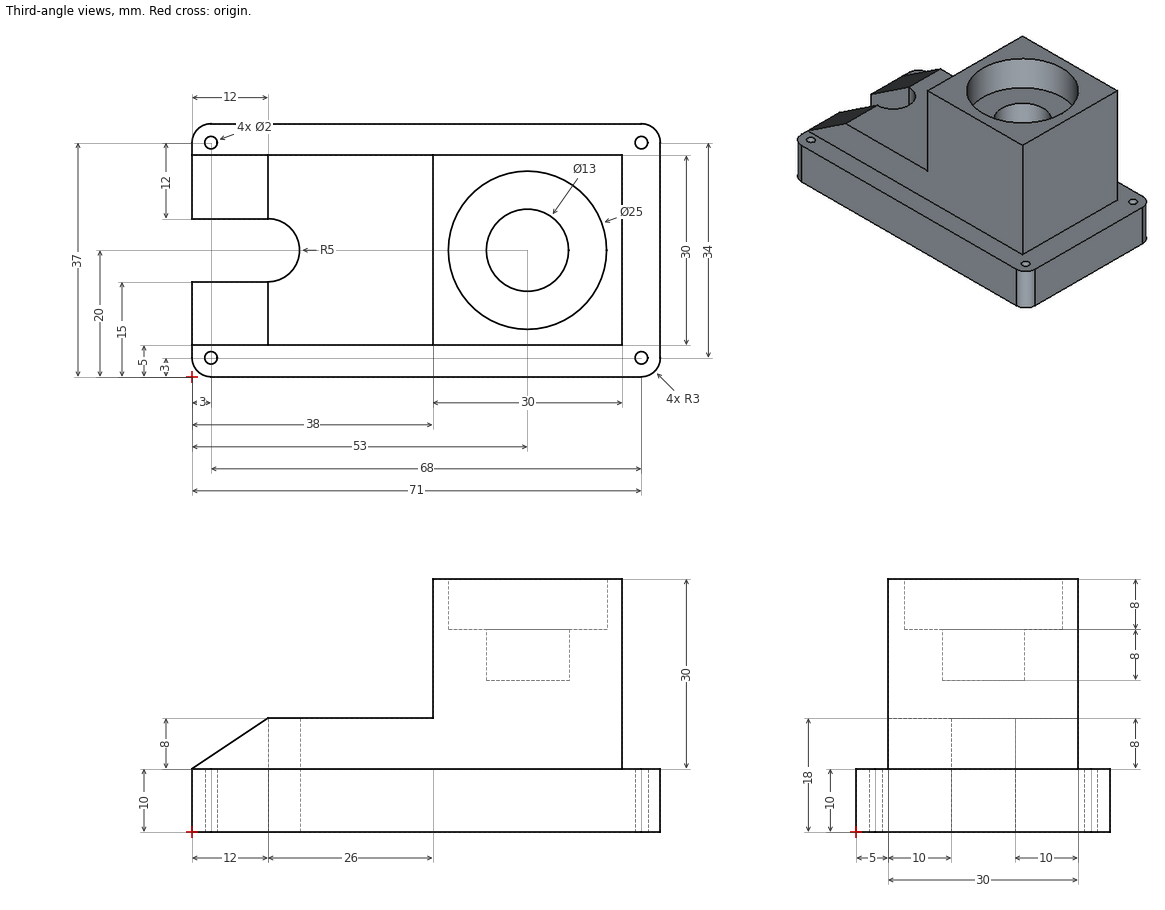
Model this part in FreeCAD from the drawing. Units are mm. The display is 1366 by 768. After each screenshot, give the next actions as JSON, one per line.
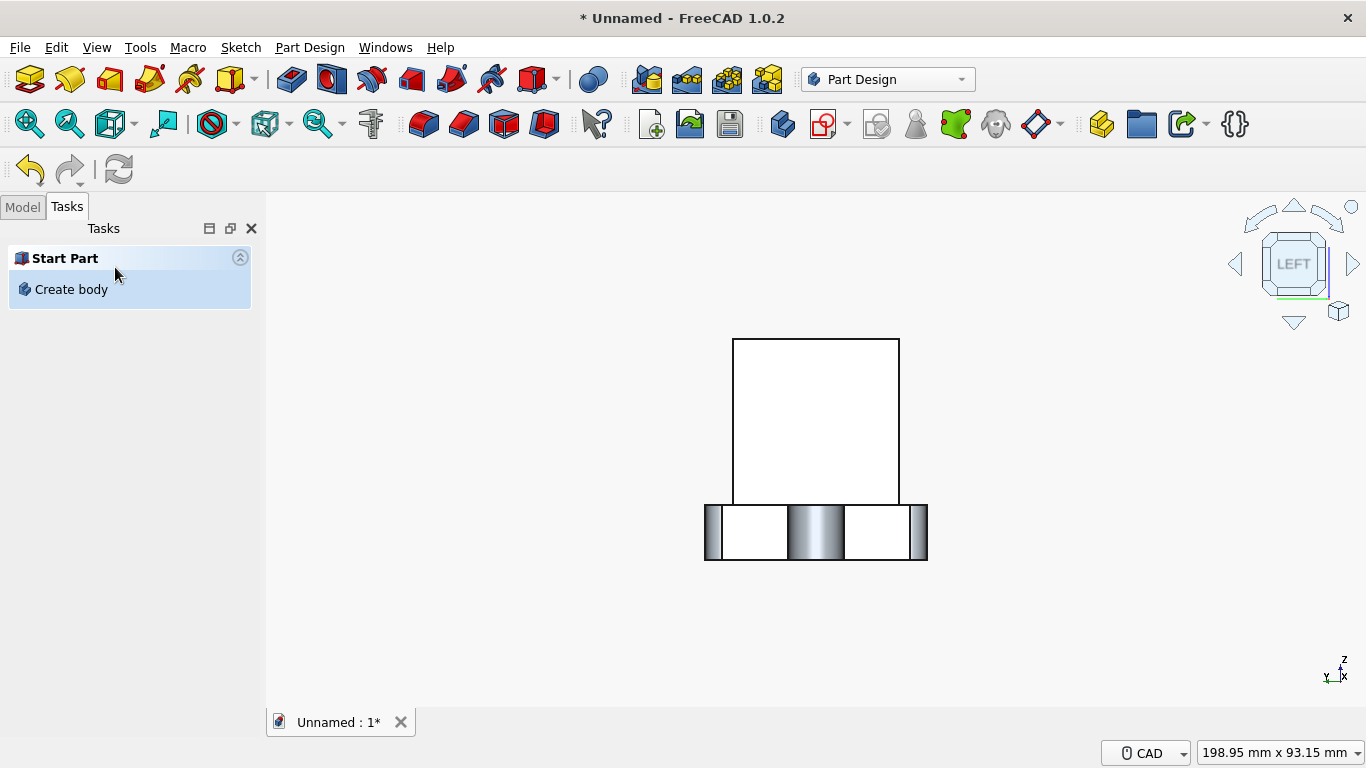
{"action": "left_click", "coordinate": [30, 124]}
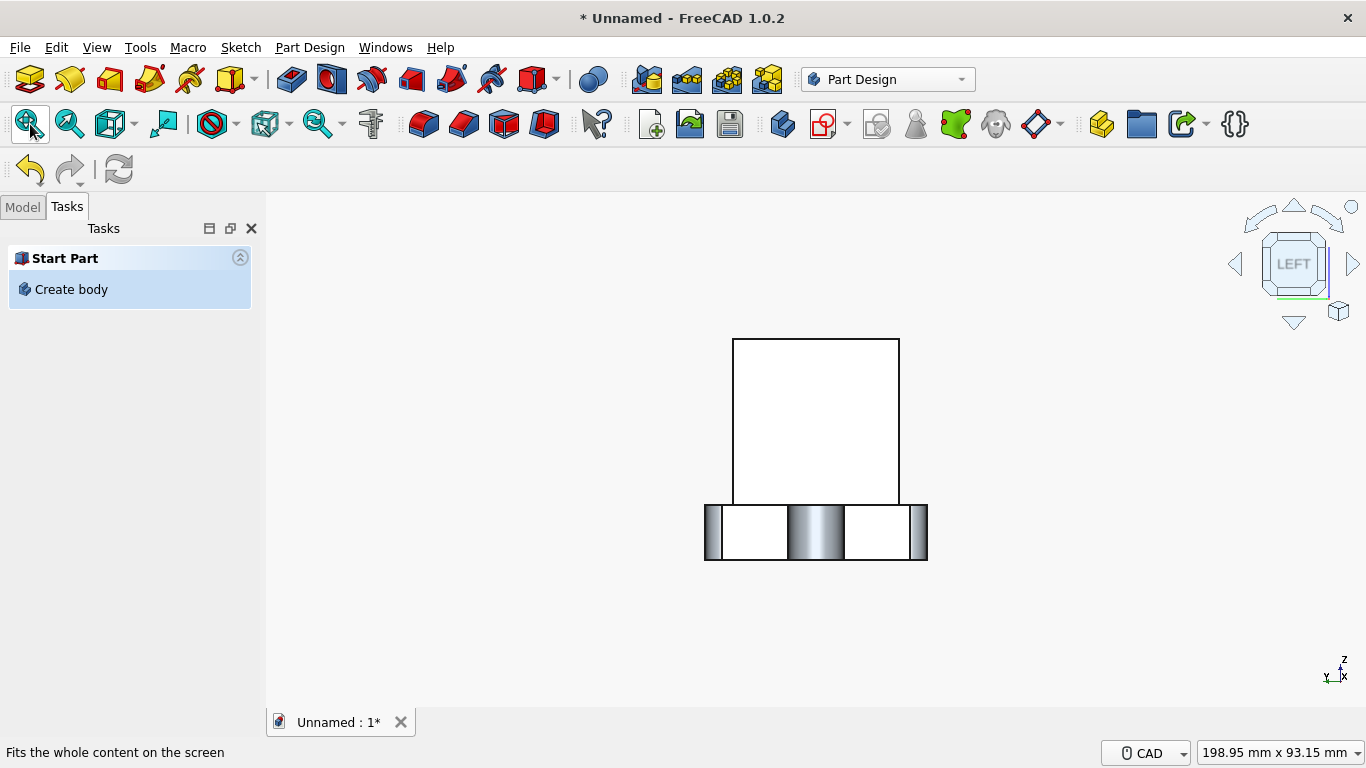
{"action": "left_click", "coordinate": [816, 421]}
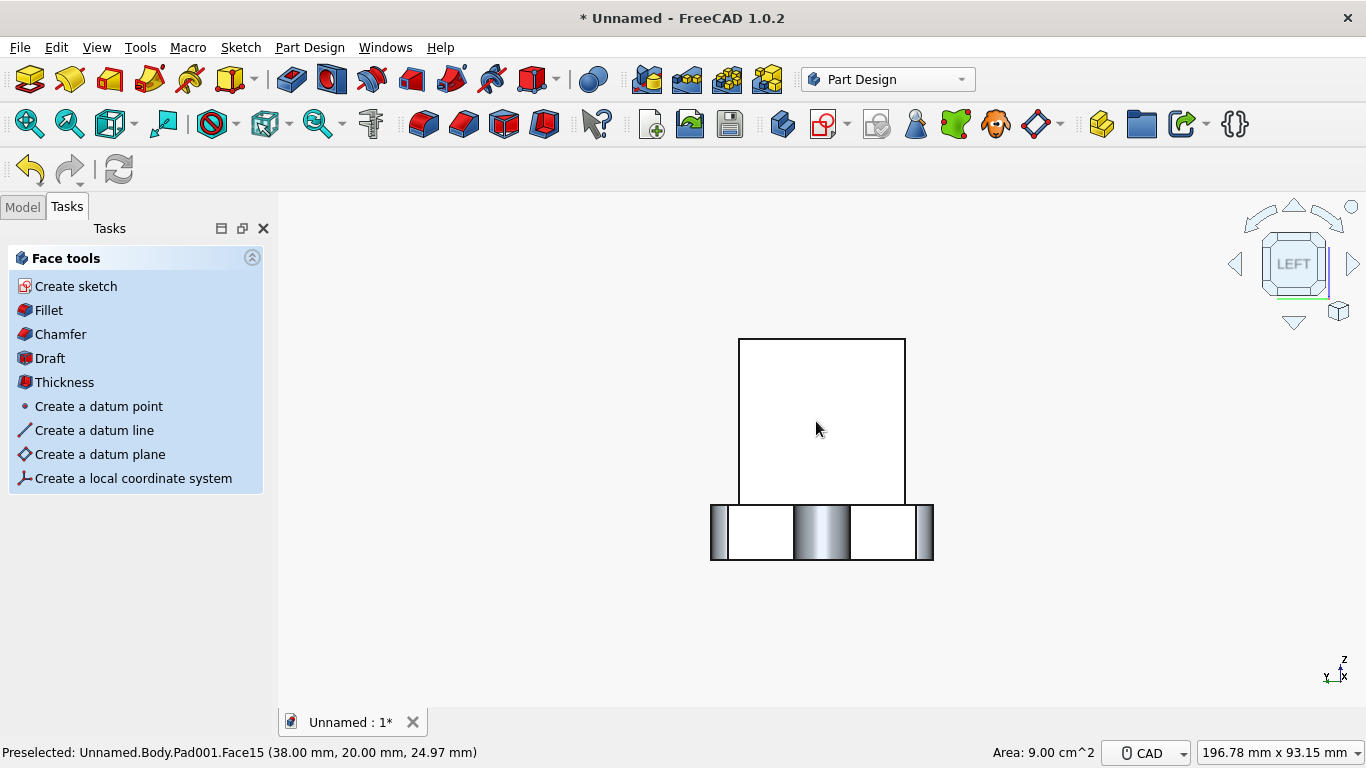
{"action": "left_click", "coordinate": [824, 124]}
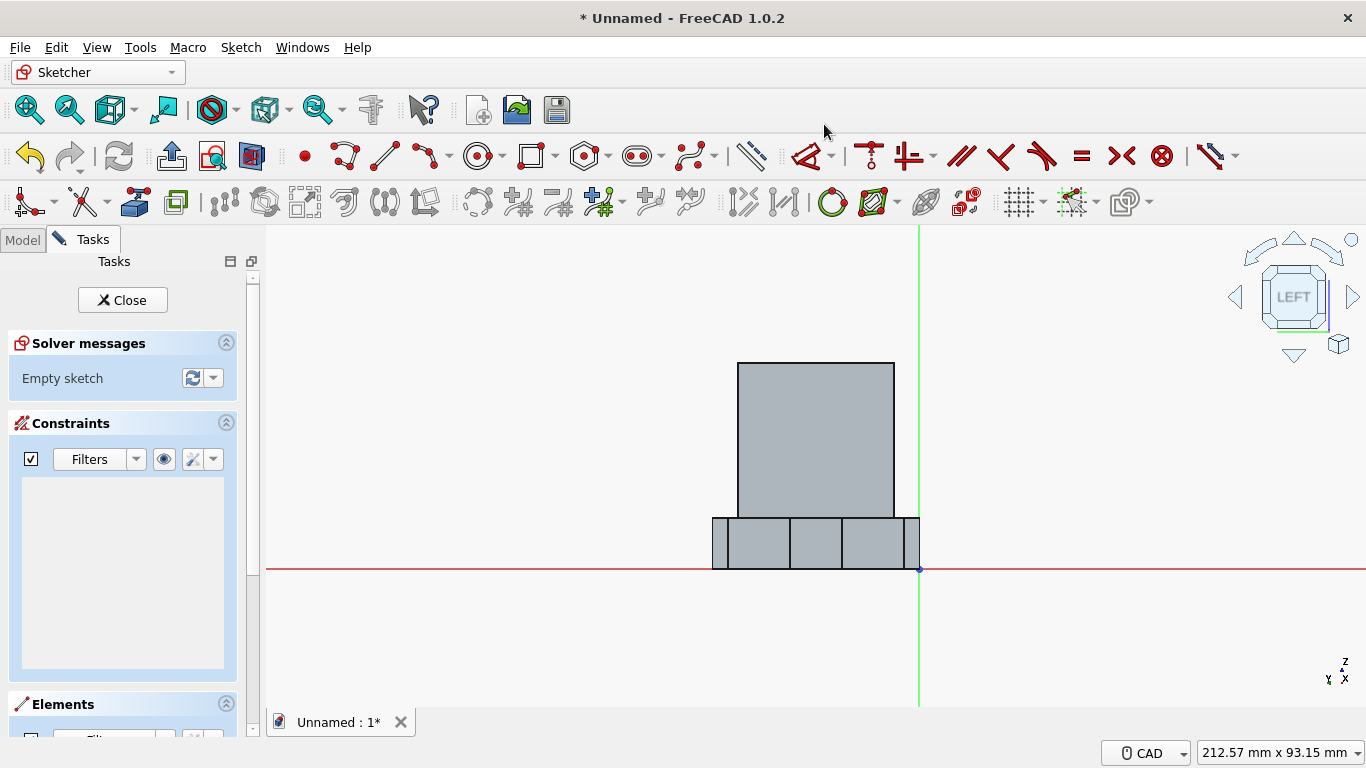
{"action": "left_click", "coordinate": [252, 156]}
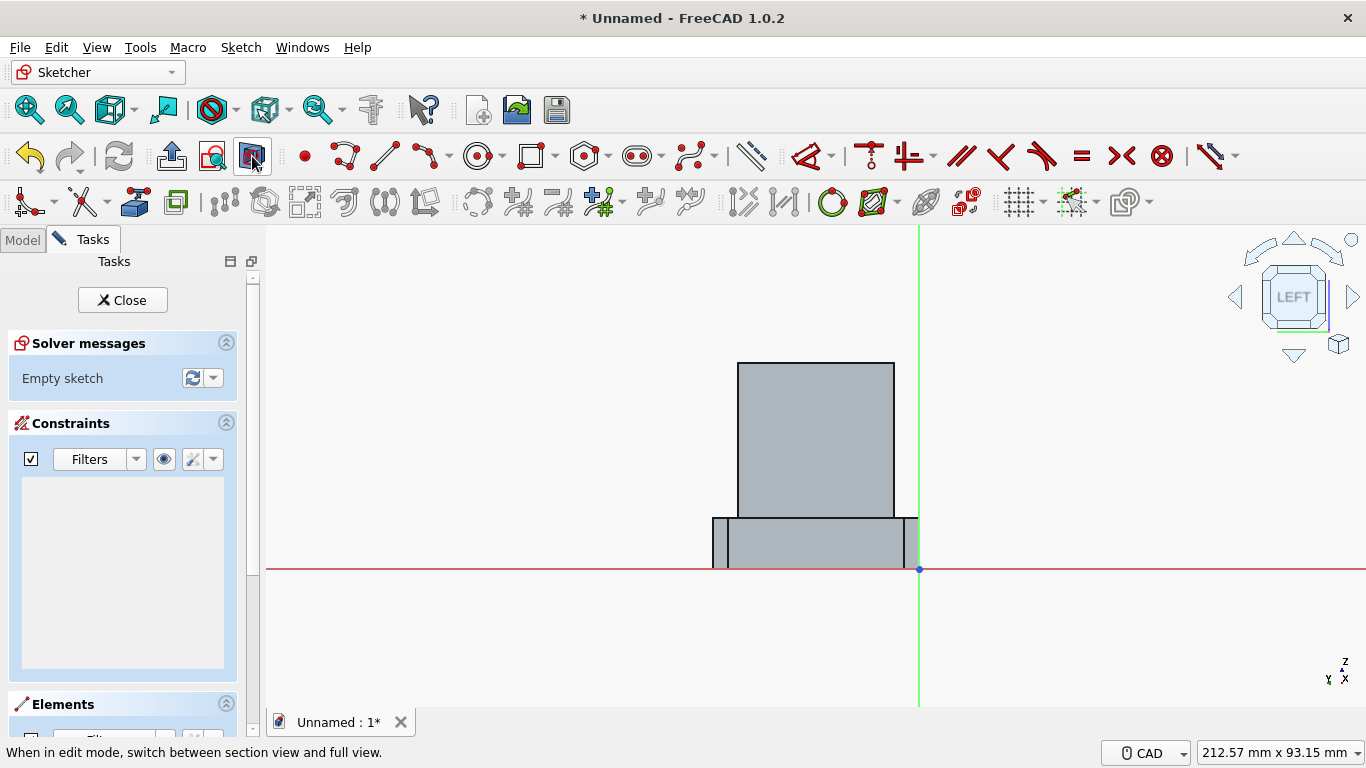
{"action": "scroll", "coordinate": [864, 547], "scroll_direction": "up", "scroll_amount": 6}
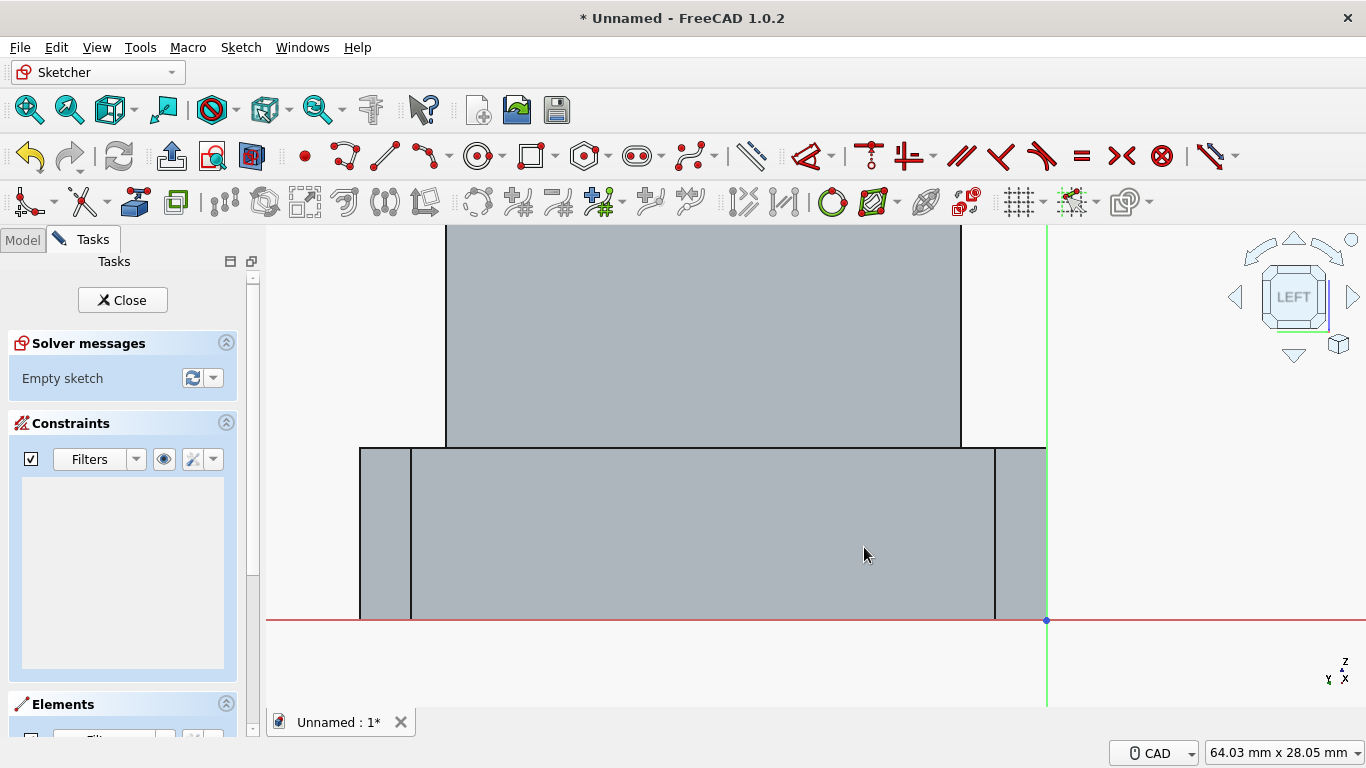
{"action": "left_click", "coordinate": [532, 156]}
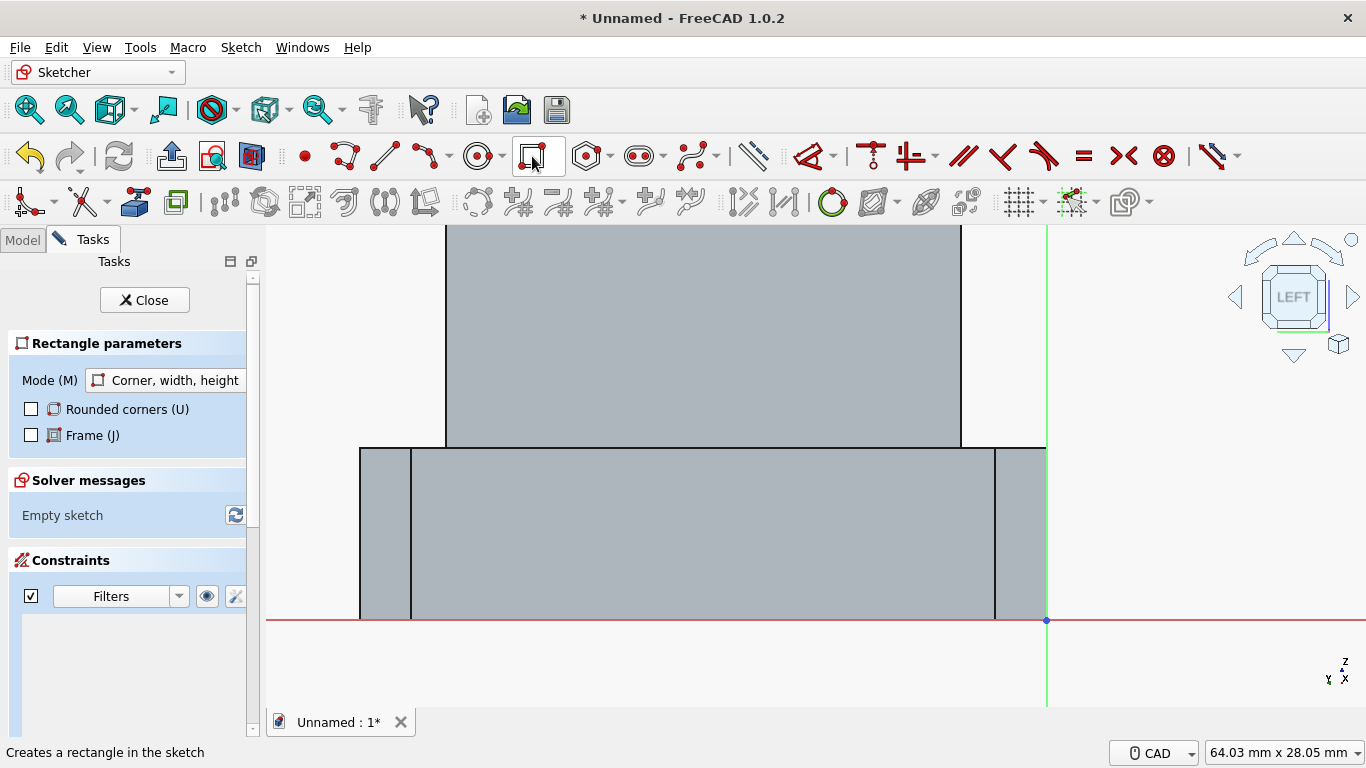
{"action": "left_click", "coordinate": [446, 311]}
{"action": "left_click", "coordinate": [961, 448]}
{"action": "key", "text": "Escape"}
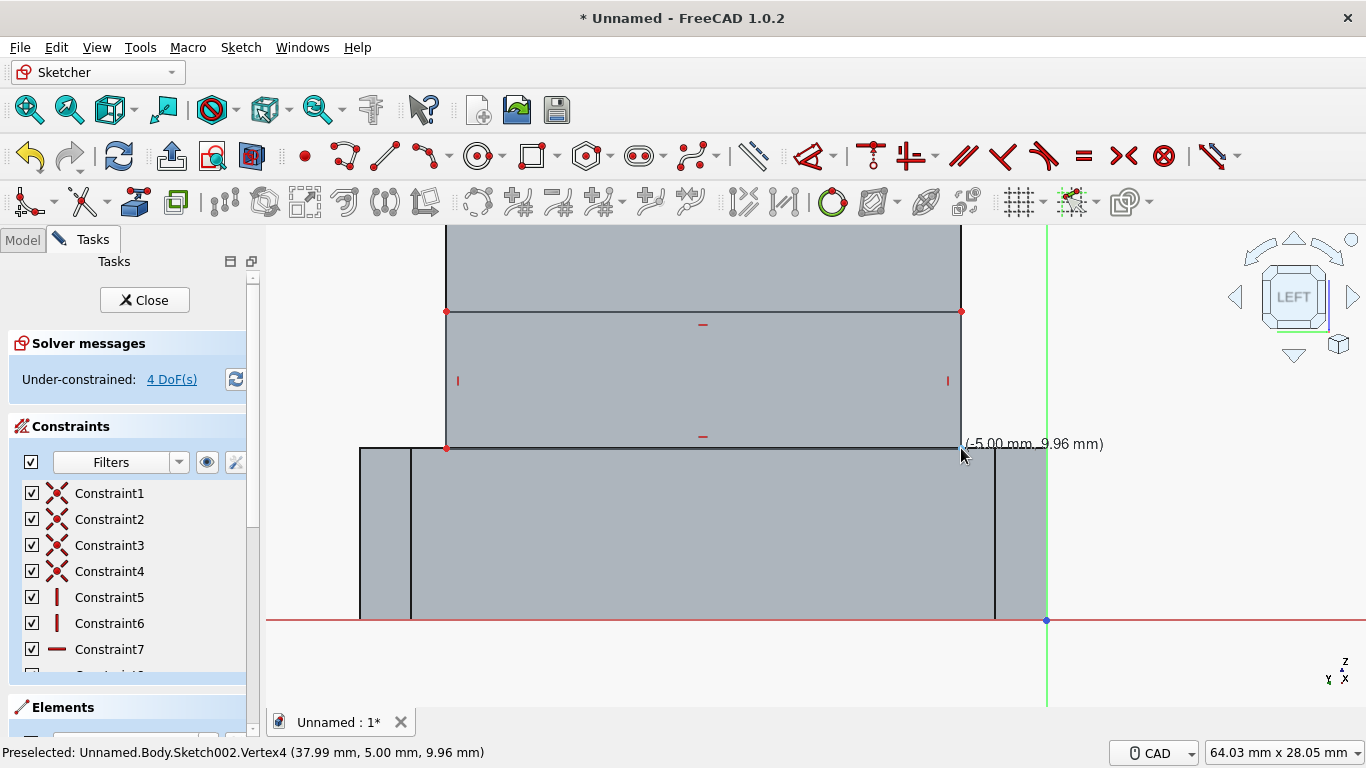
{"action": "left_click", "coordinate": [808, 156]}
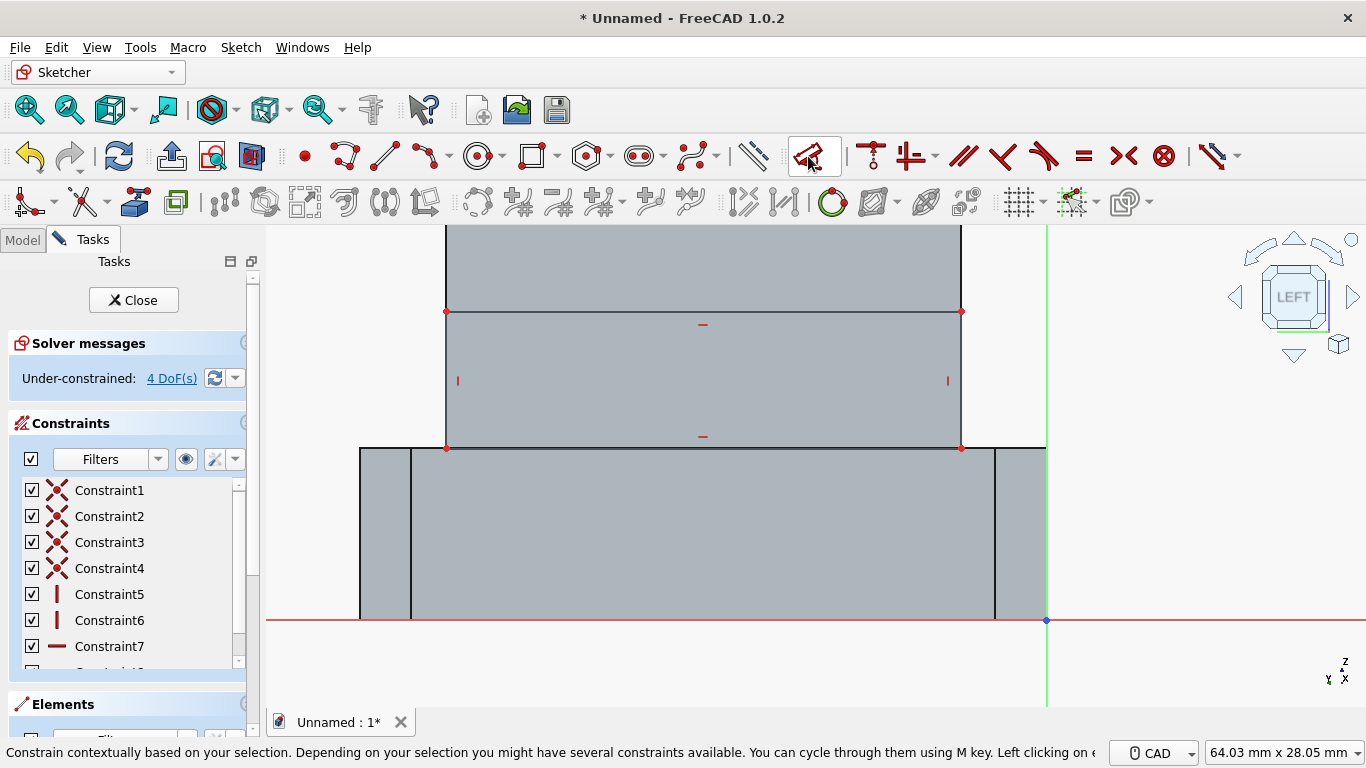
{"action": "left_click", "coordinate": [446, 353]}
{"action": "left_click", "coordinate": [412, 380]}